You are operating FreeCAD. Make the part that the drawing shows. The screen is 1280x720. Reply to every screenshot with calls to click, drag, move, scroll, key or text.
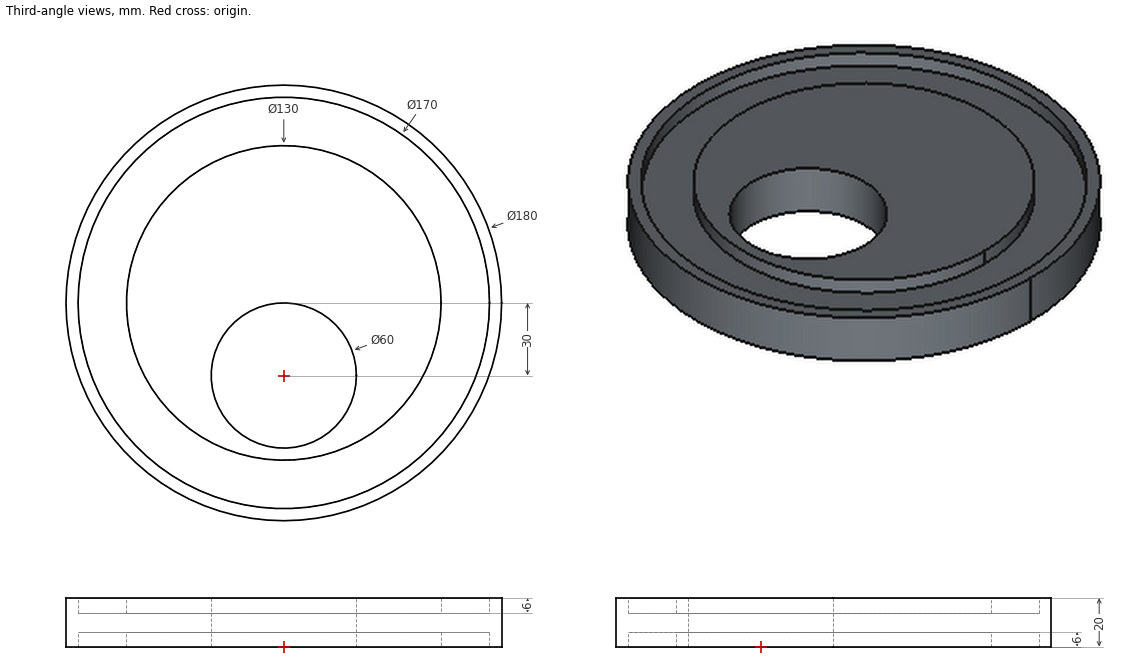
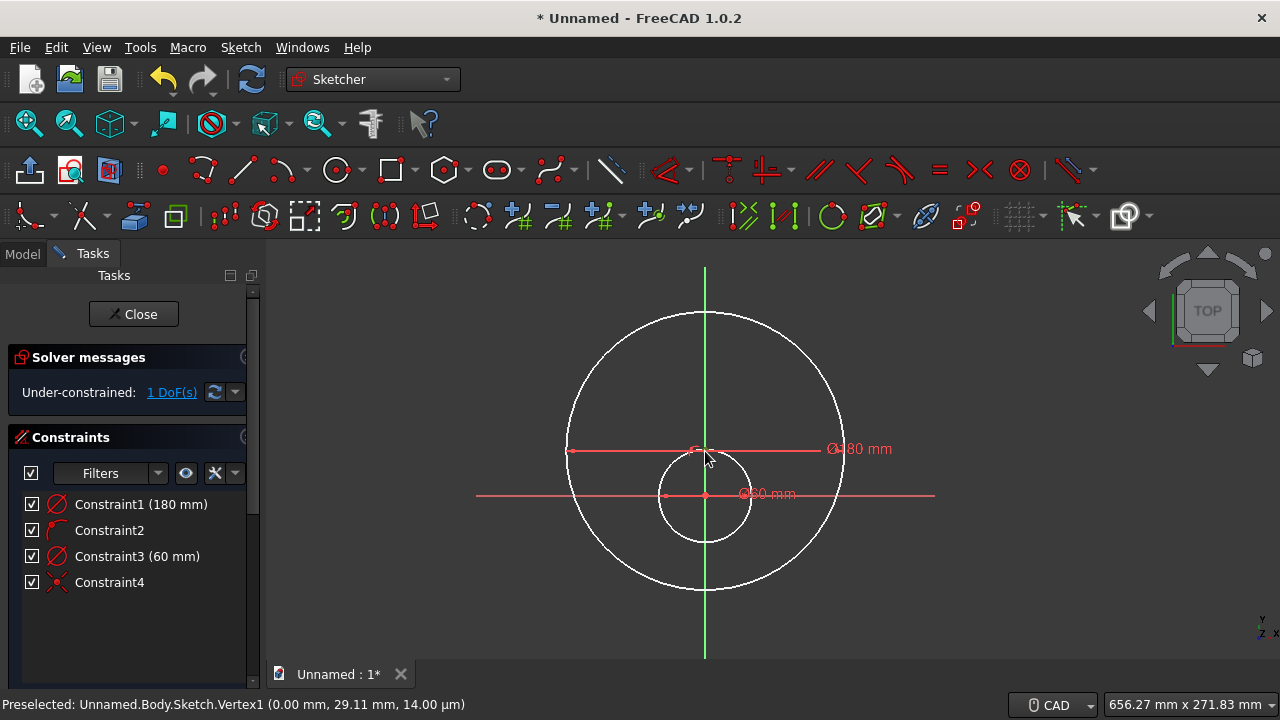
click(692, 170)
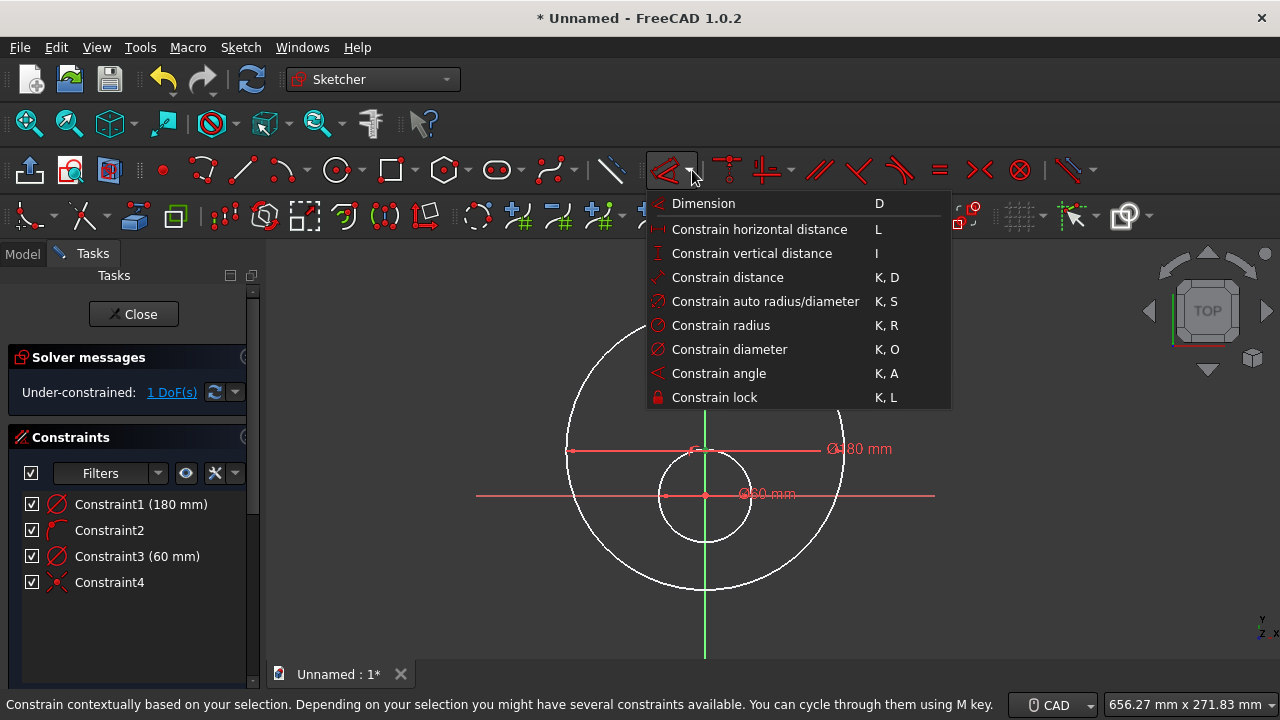
click(799, 253)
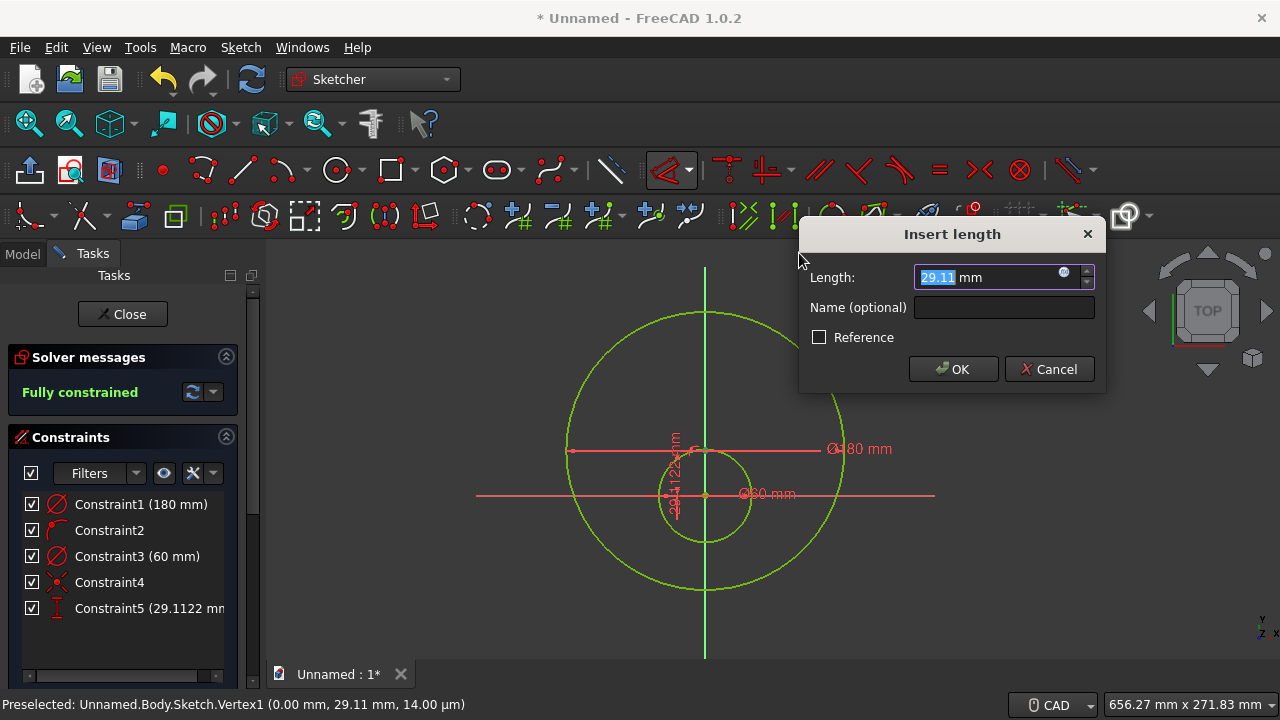
text(30)
key(Return)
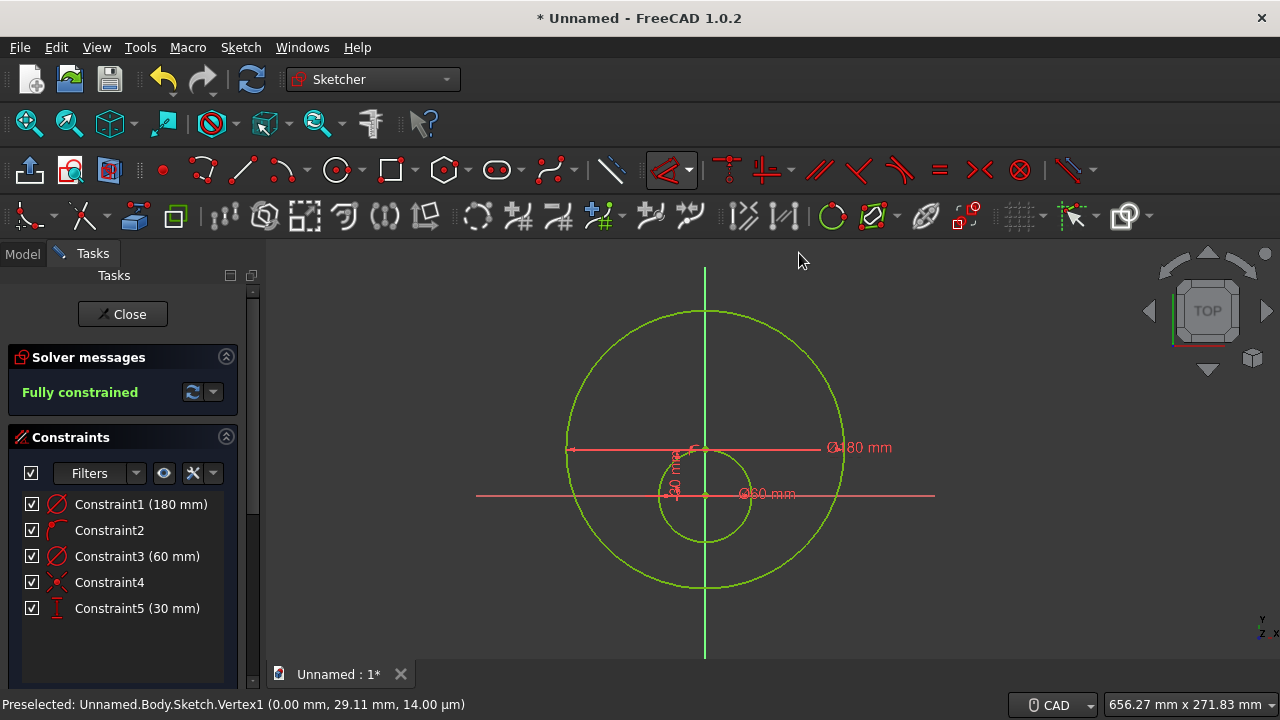
click(123, 314)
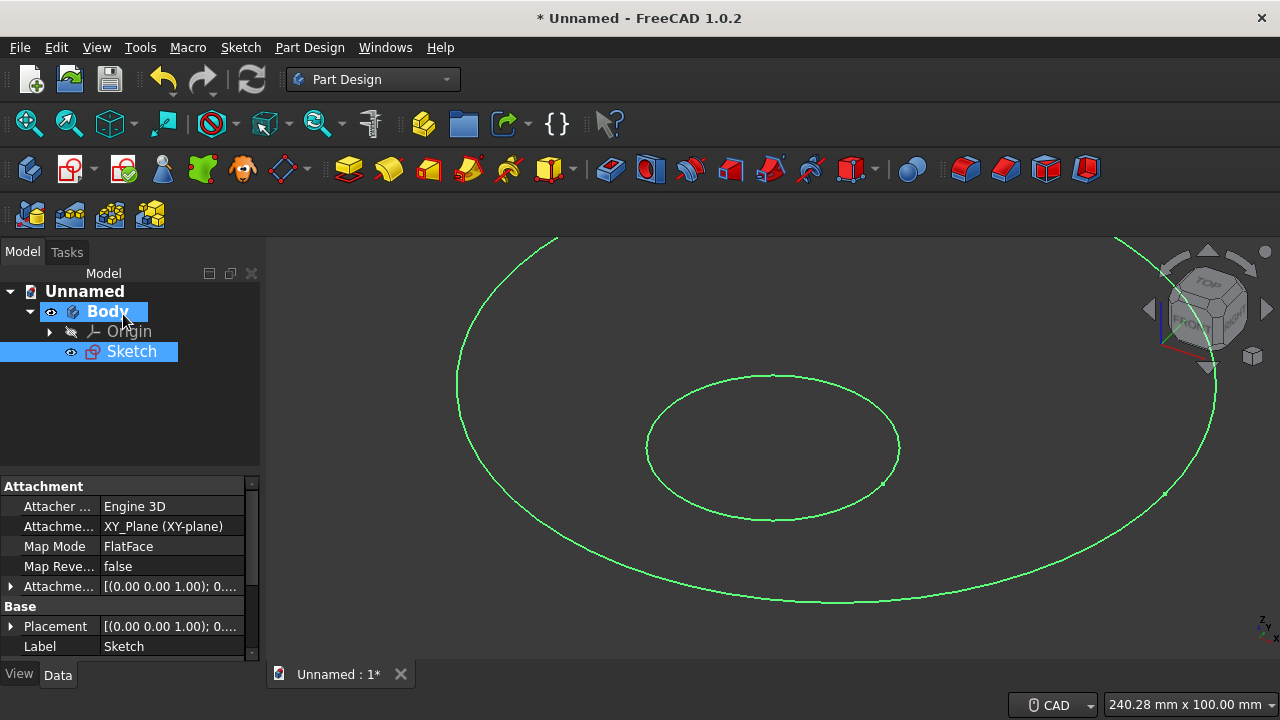
click(350, 170)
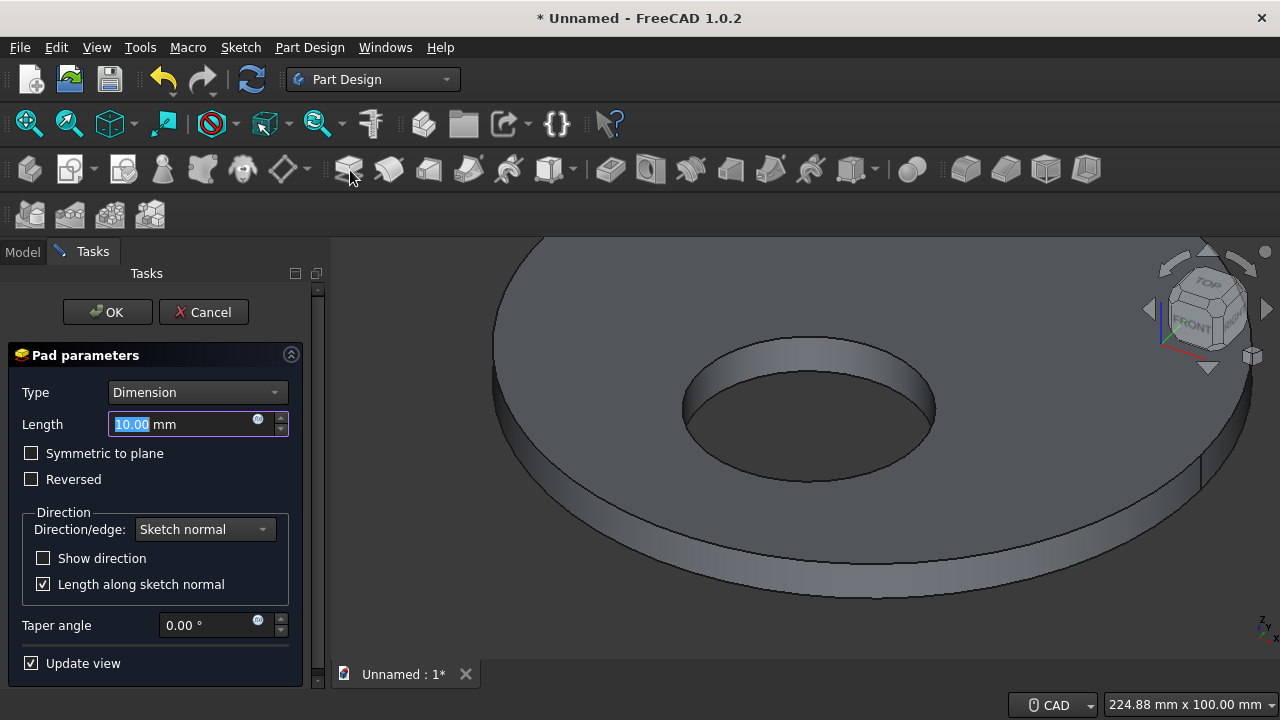
text(20)
key(Tab)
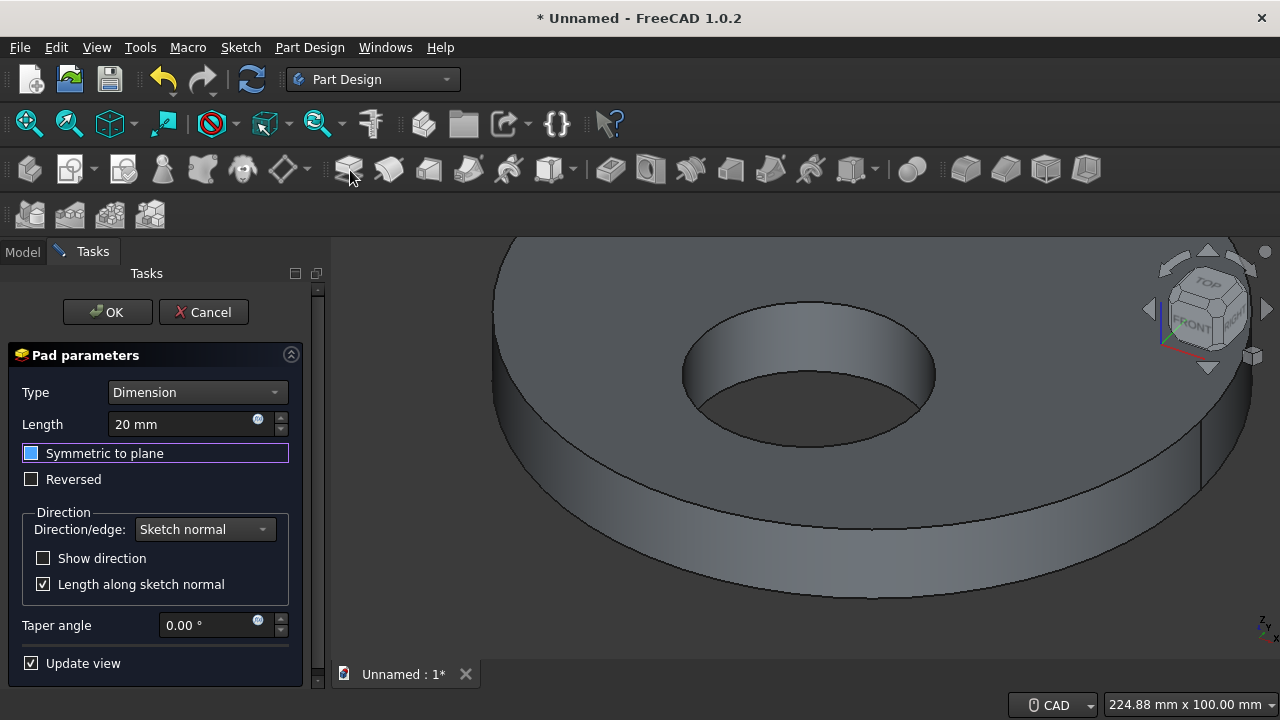
click(108, 312)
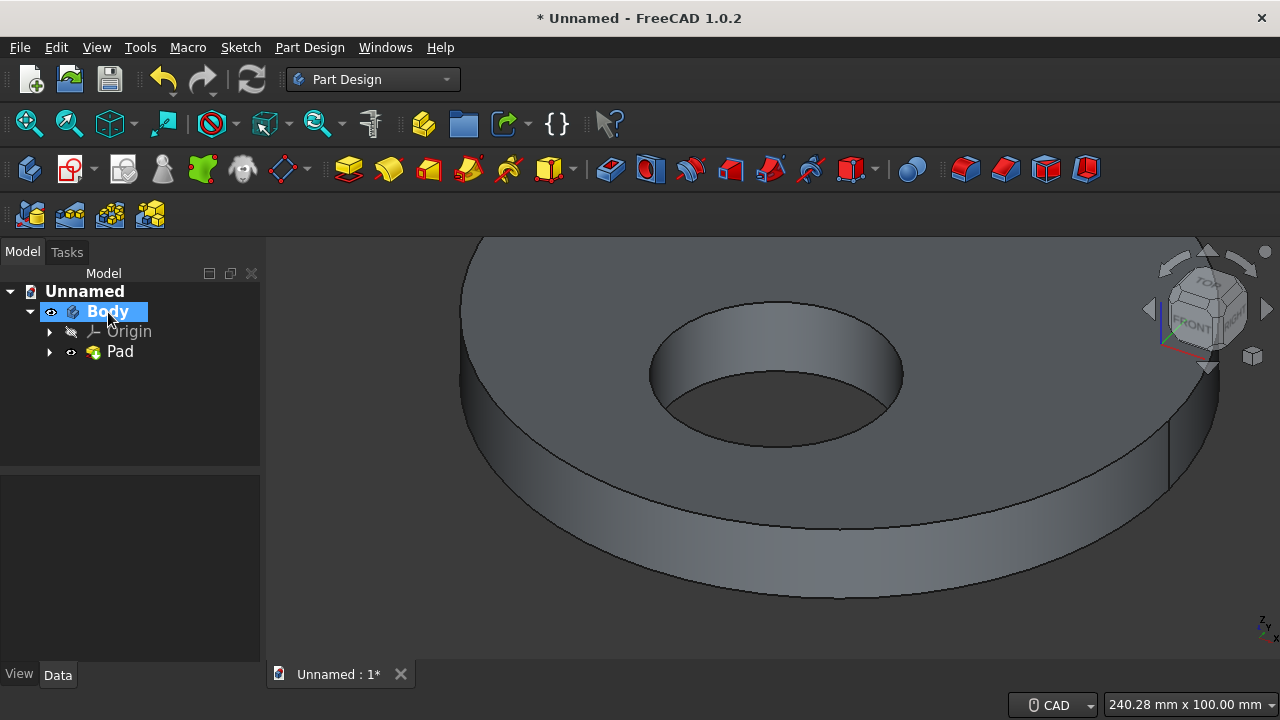
click(30, 124)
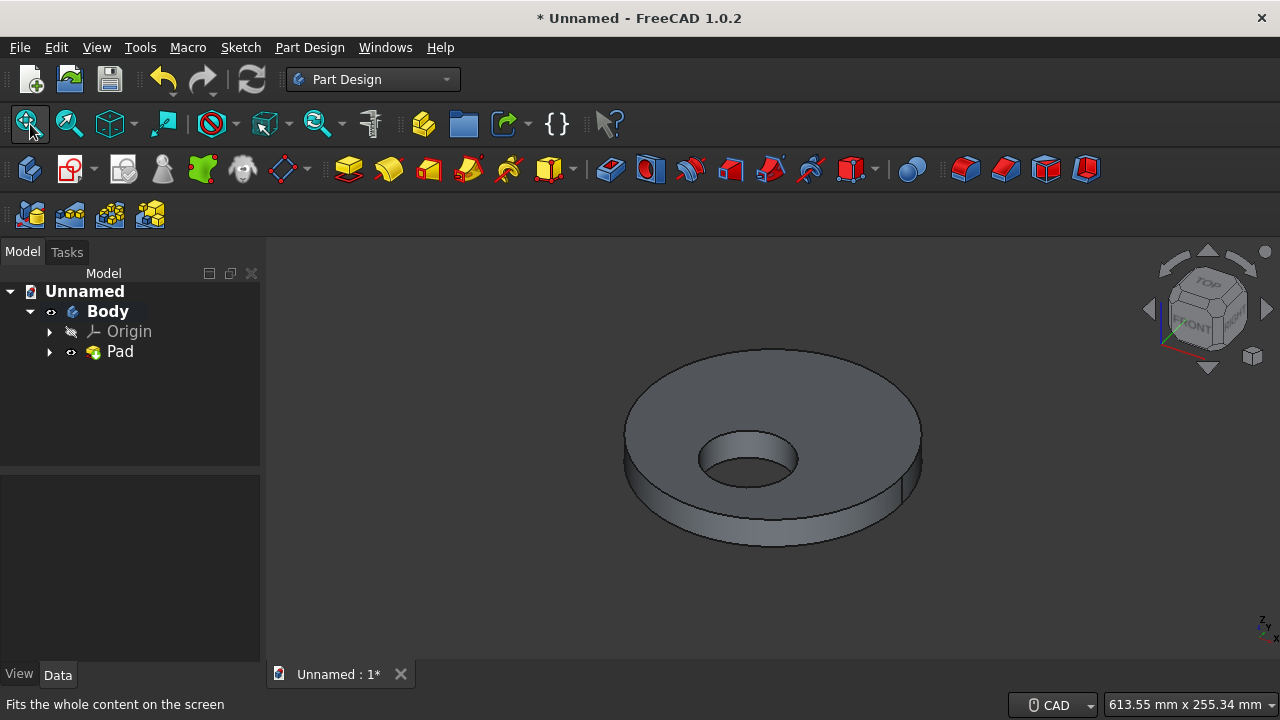
click(815, 391)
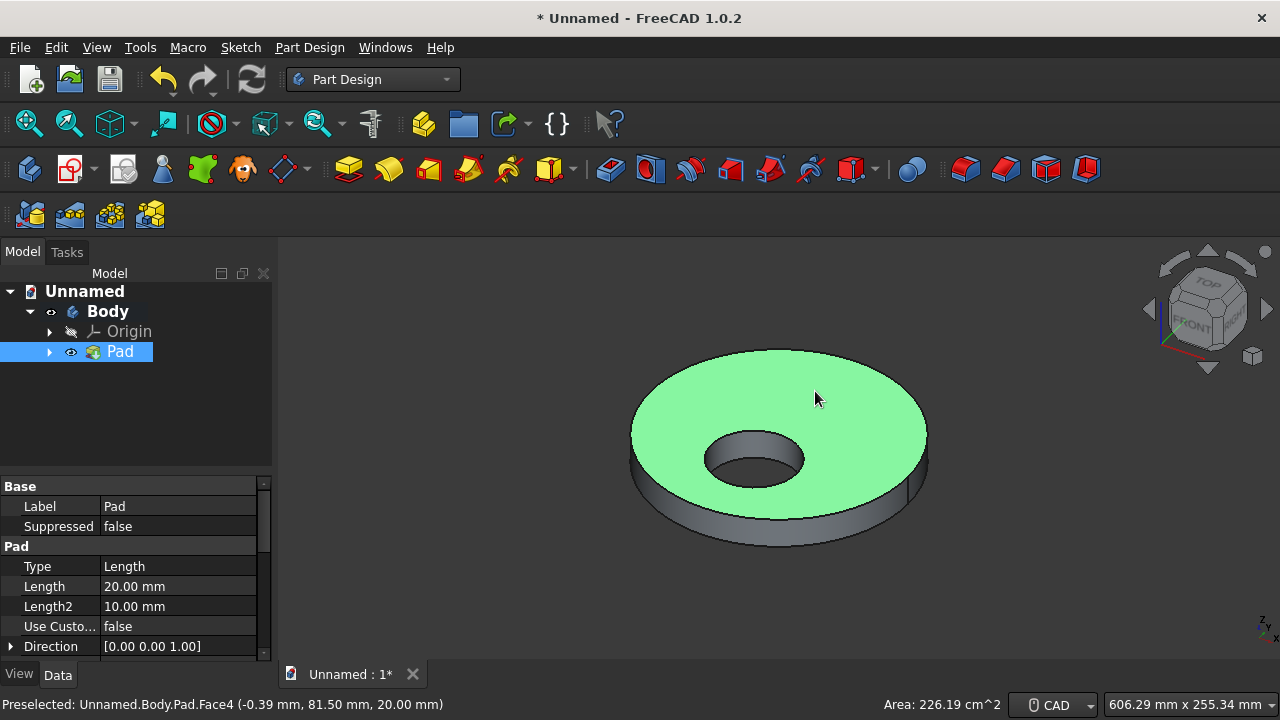
click(70, 170)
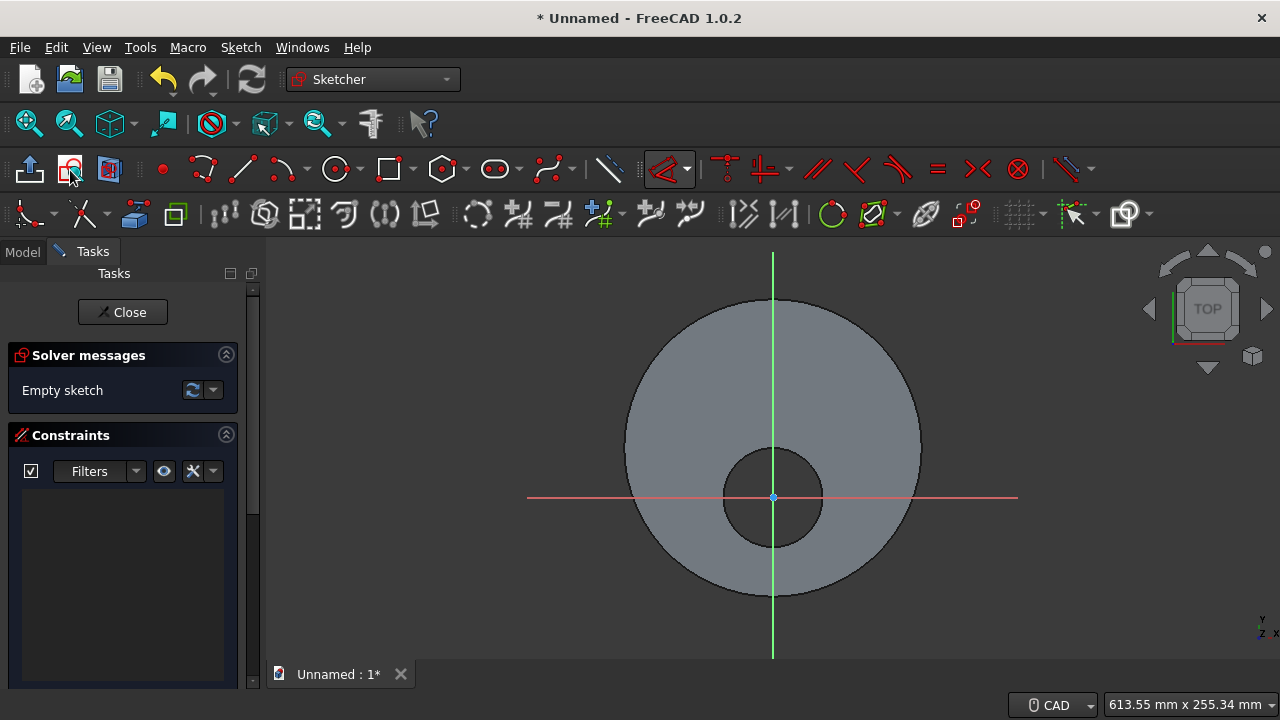
click(336, 170)